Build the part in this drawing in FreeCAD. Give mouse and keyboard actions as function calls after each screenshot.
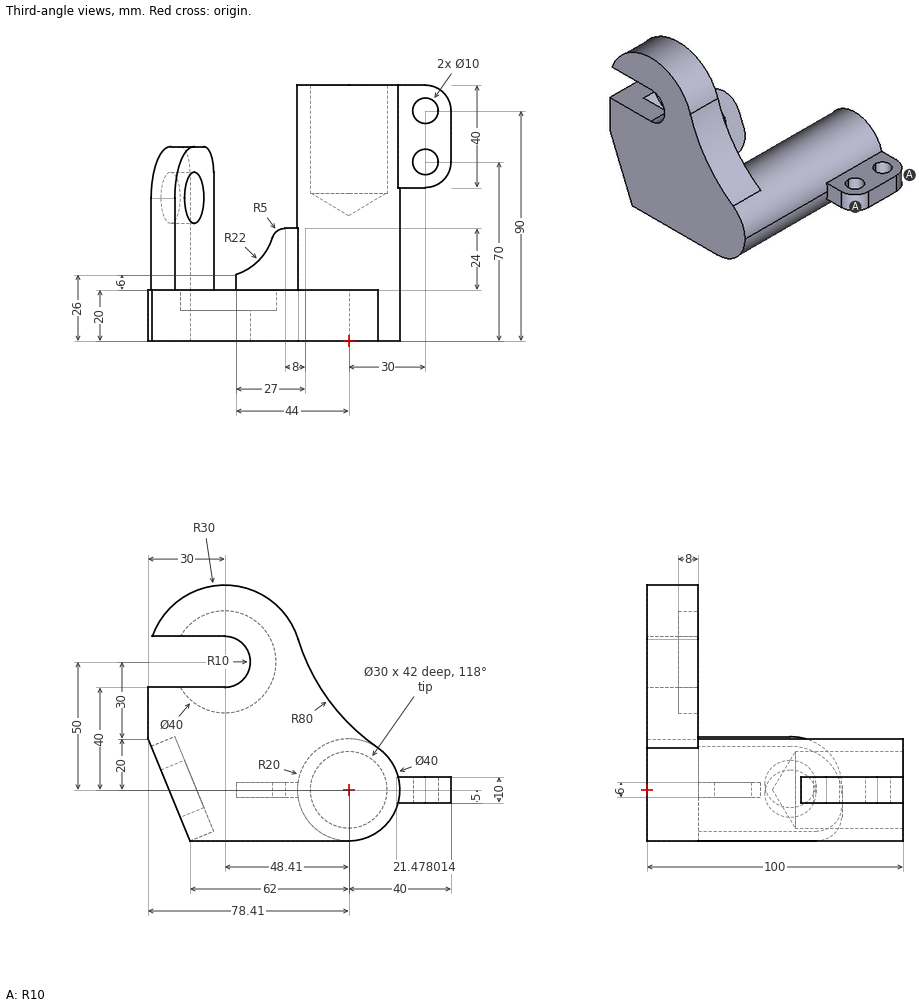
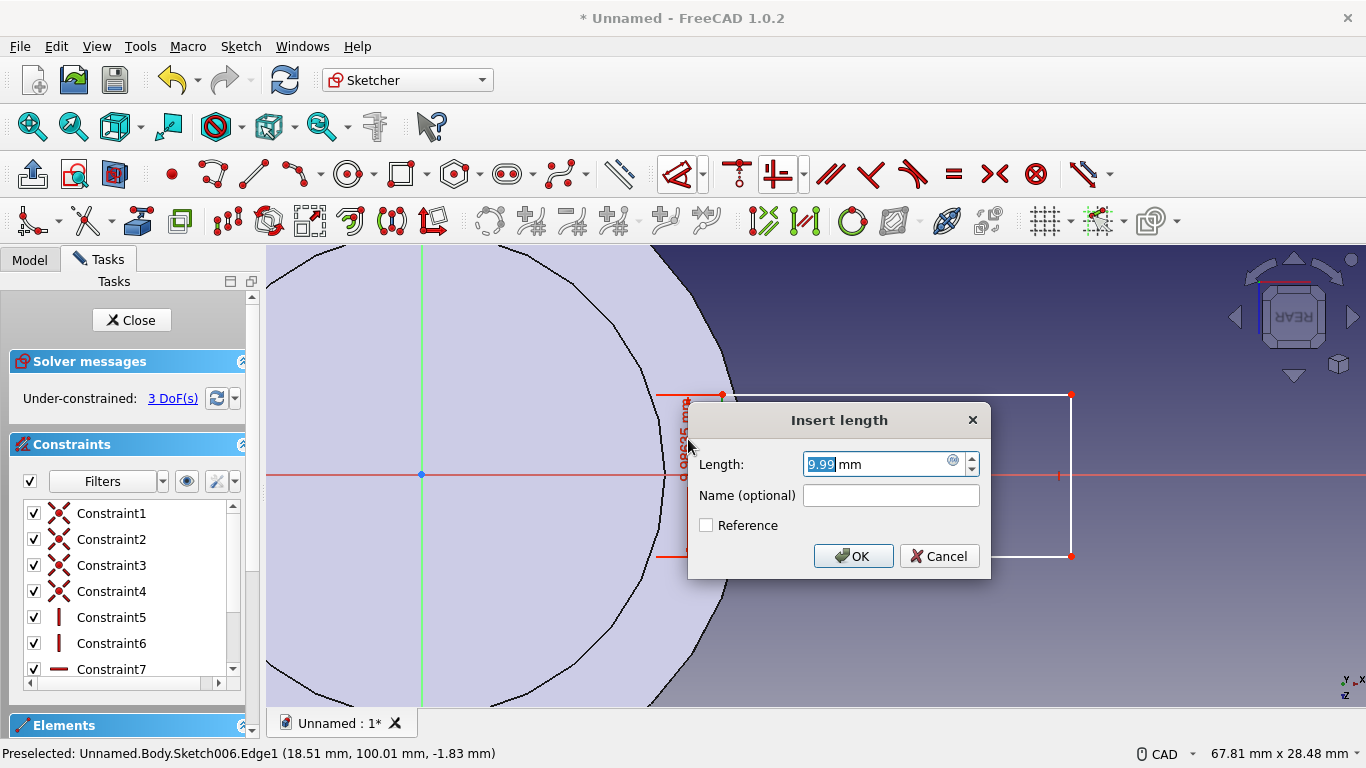
text(10)
key(Return)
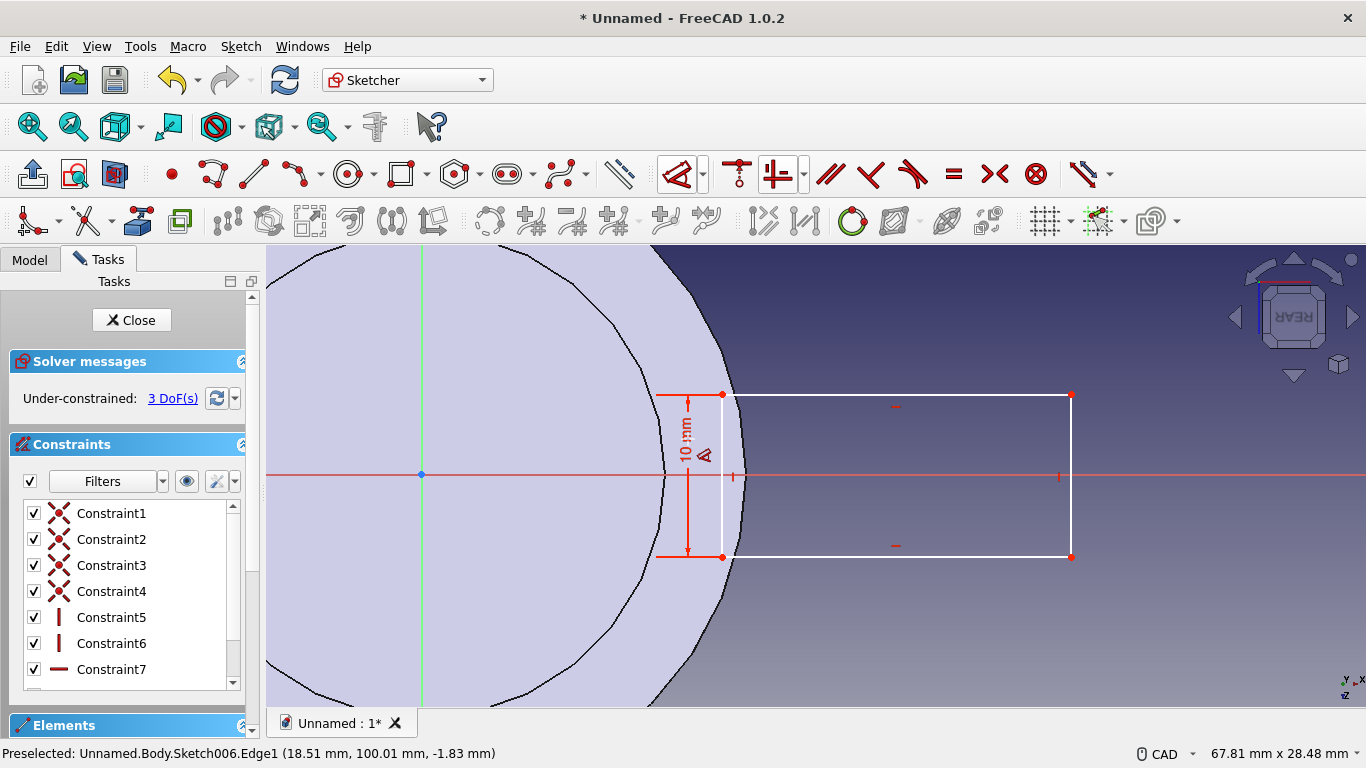
click(722, 395)
click(388, 435)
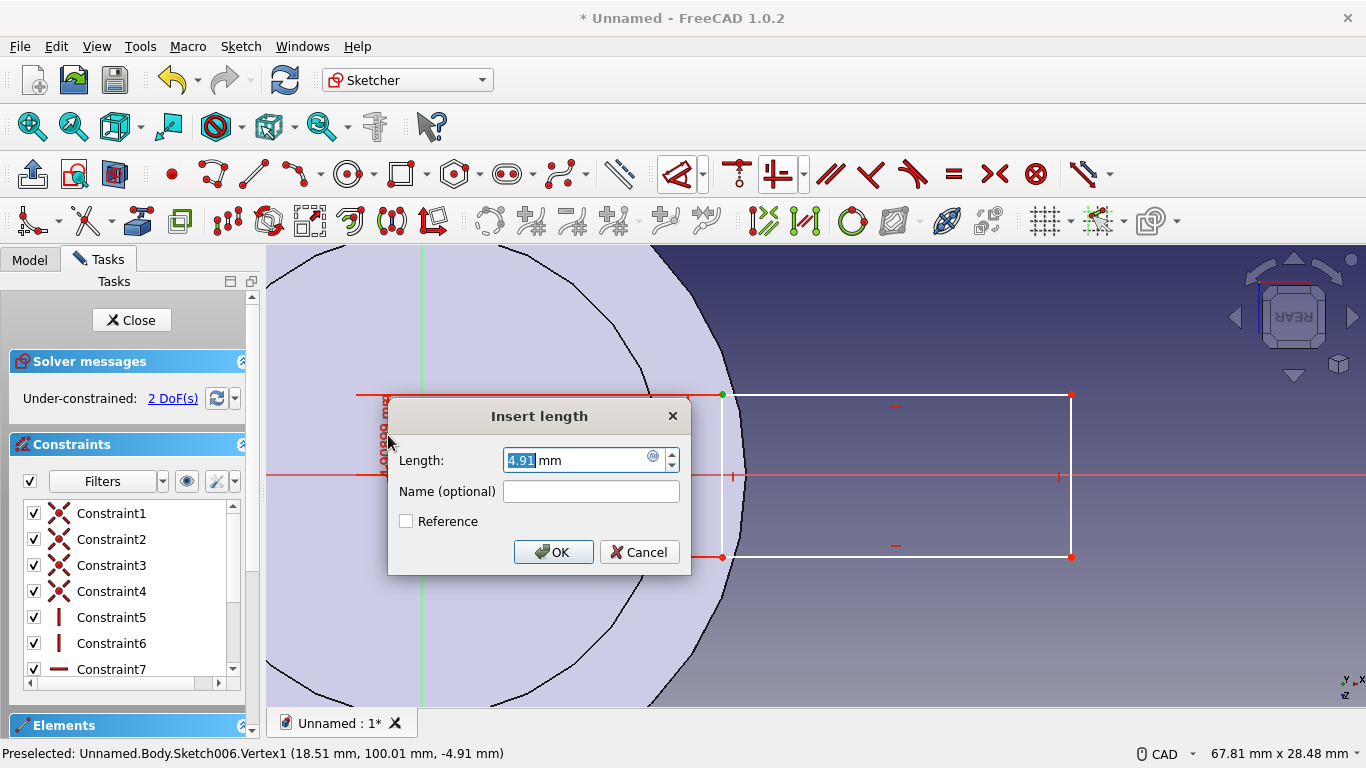
text(5)
key(Return)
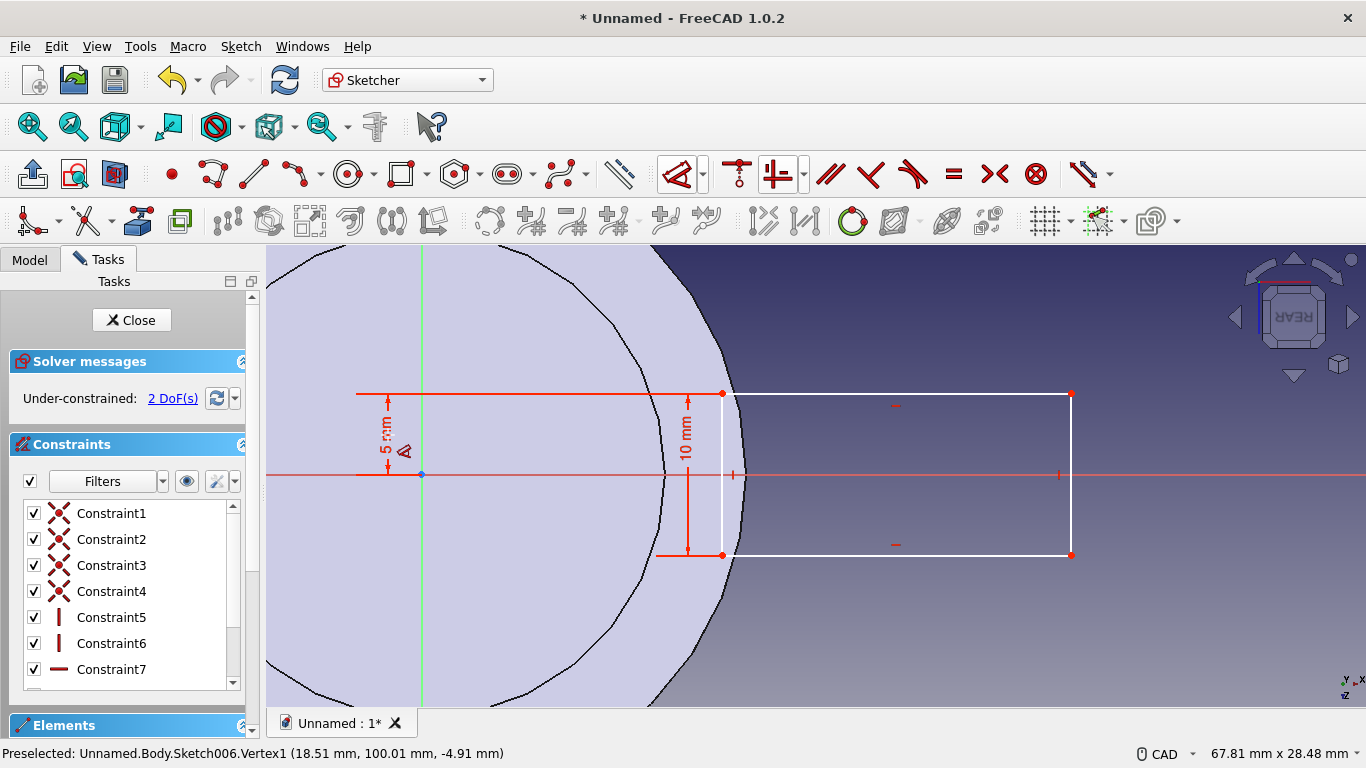
click(1071, 556)
click(746, 590)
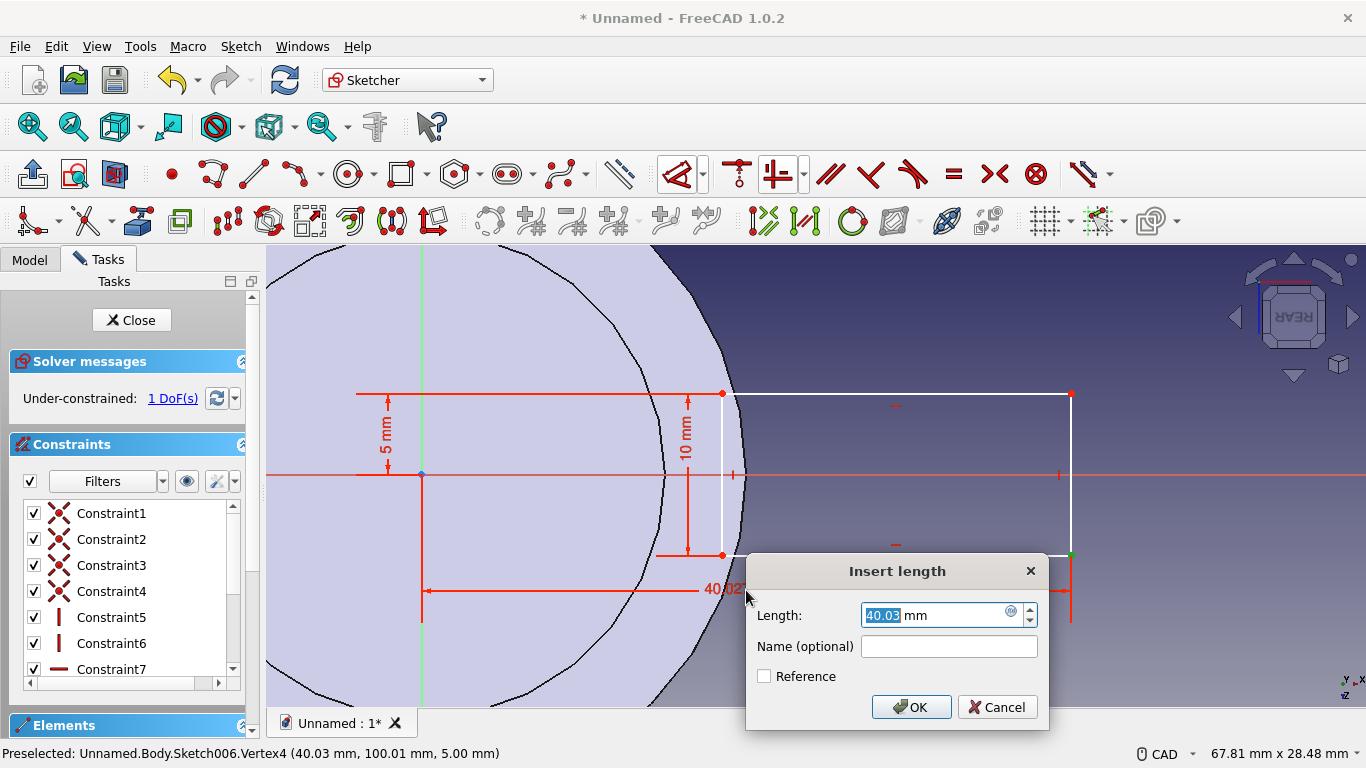
text(40)
key(Return)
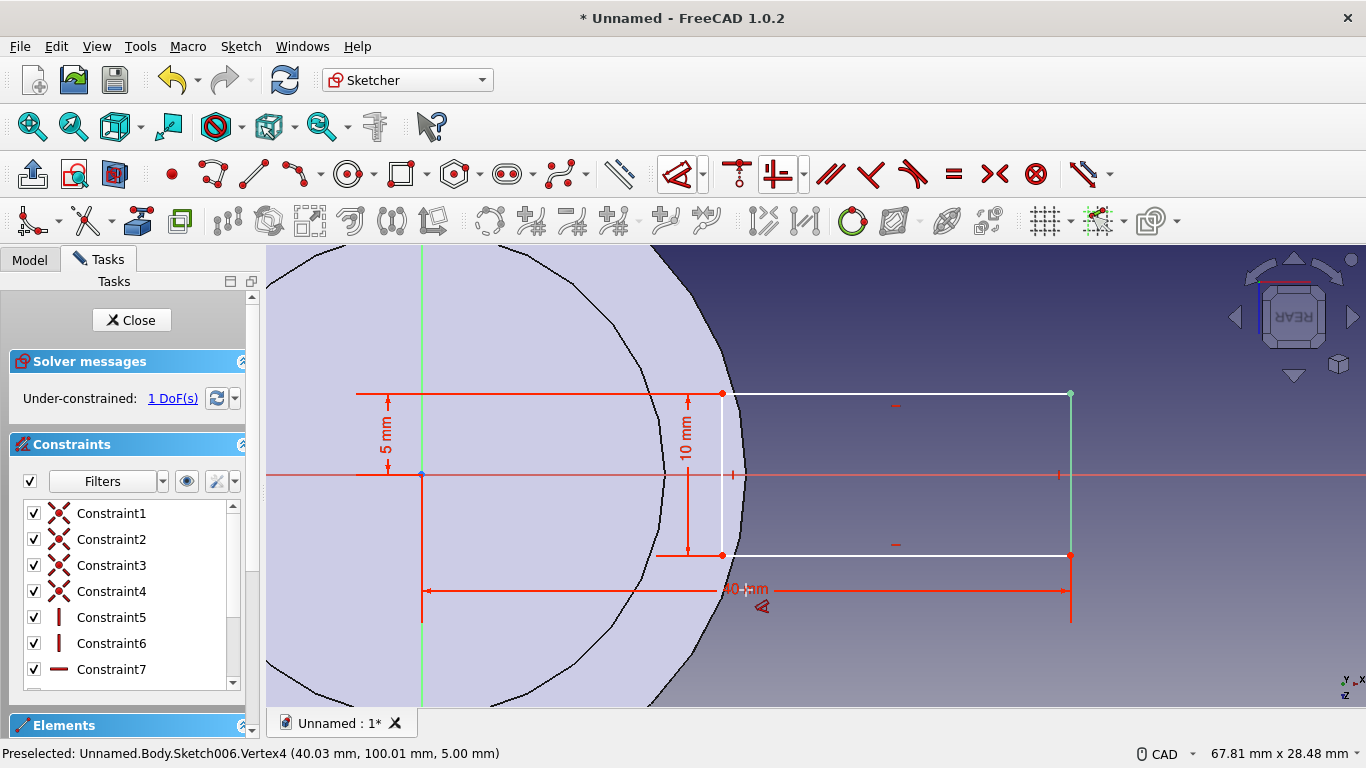
click(827, 556)
click(896, 590)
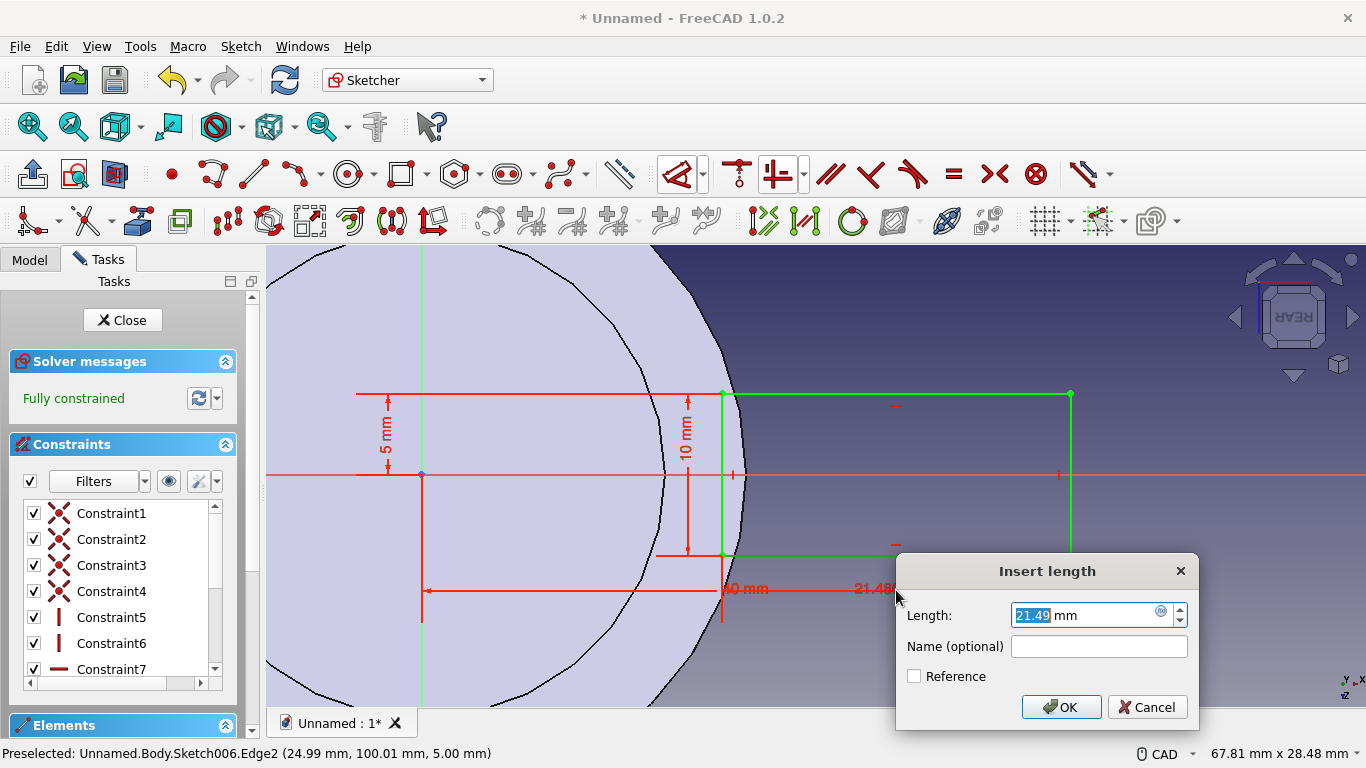
text(21.478014)
key(Return)
key(Escape)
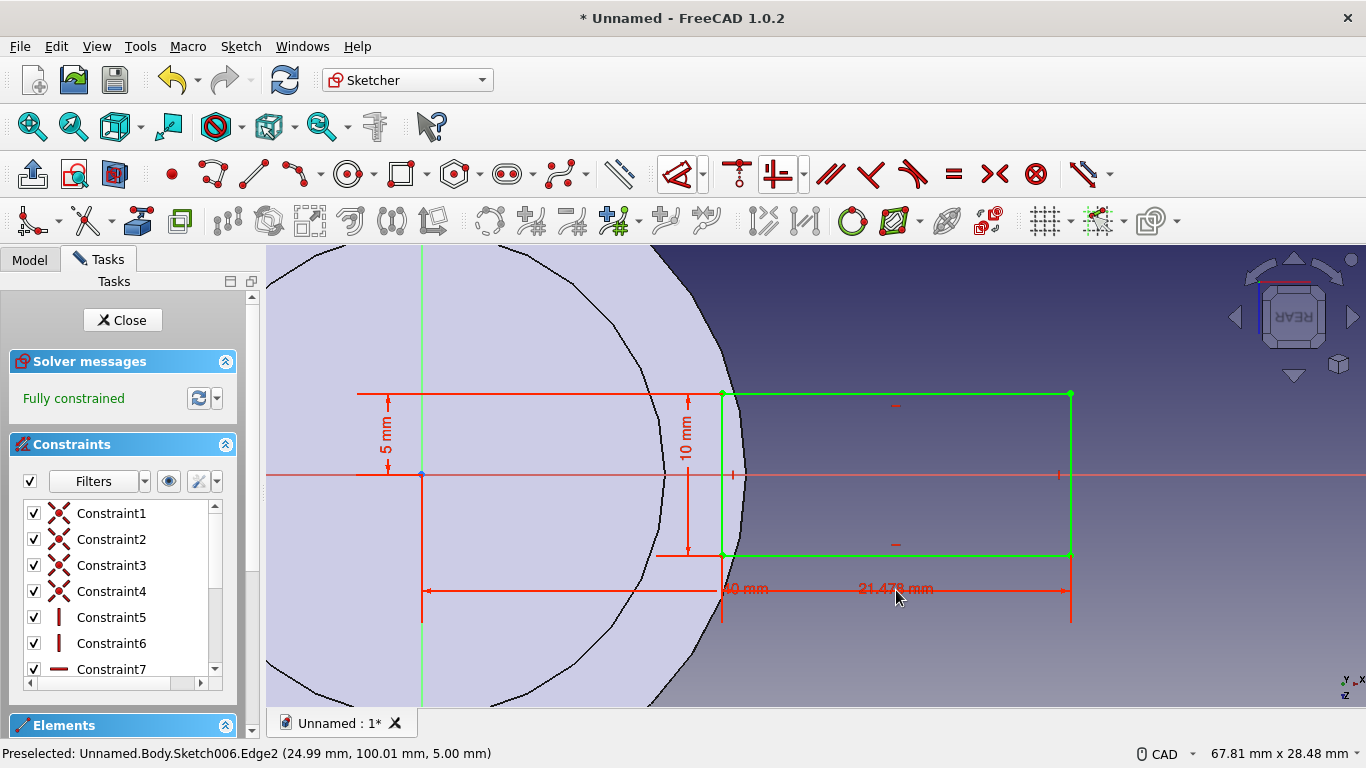
click(123, 320)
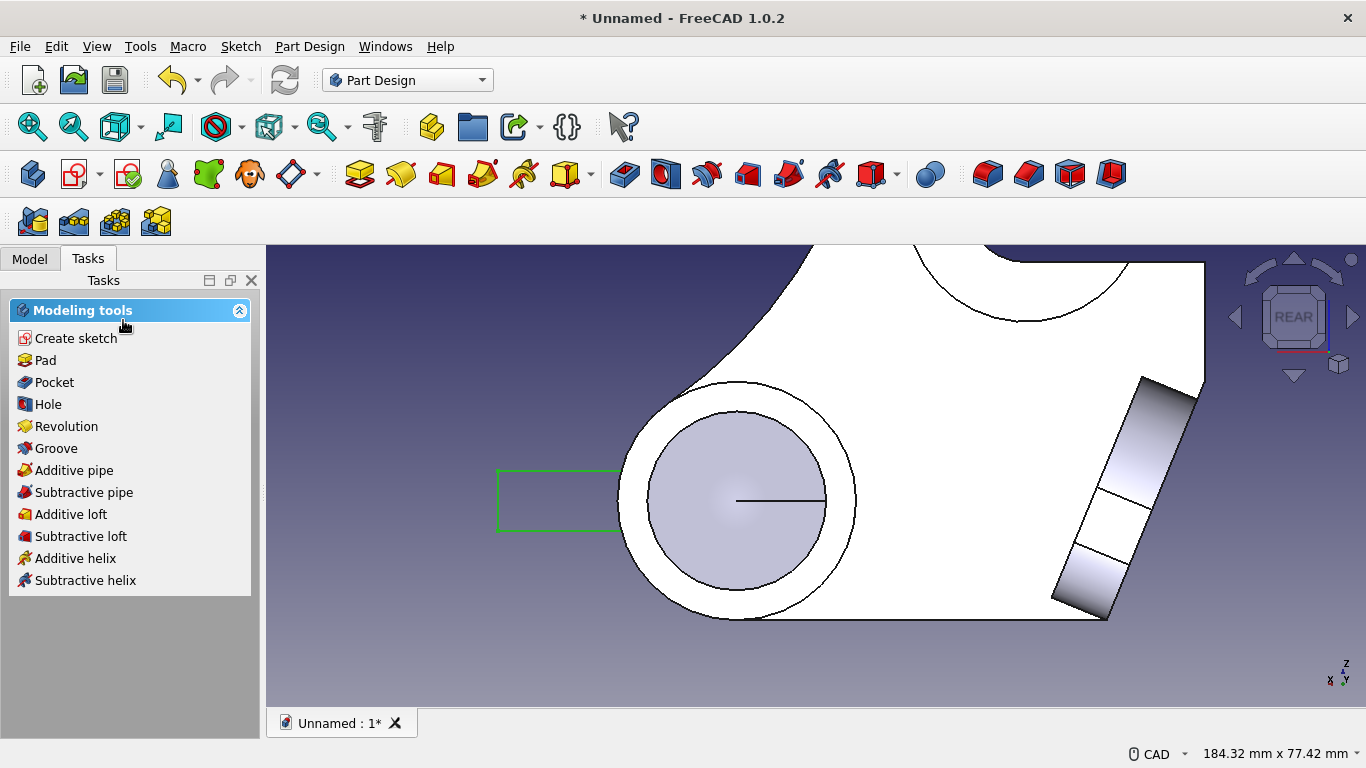
click(360, 174)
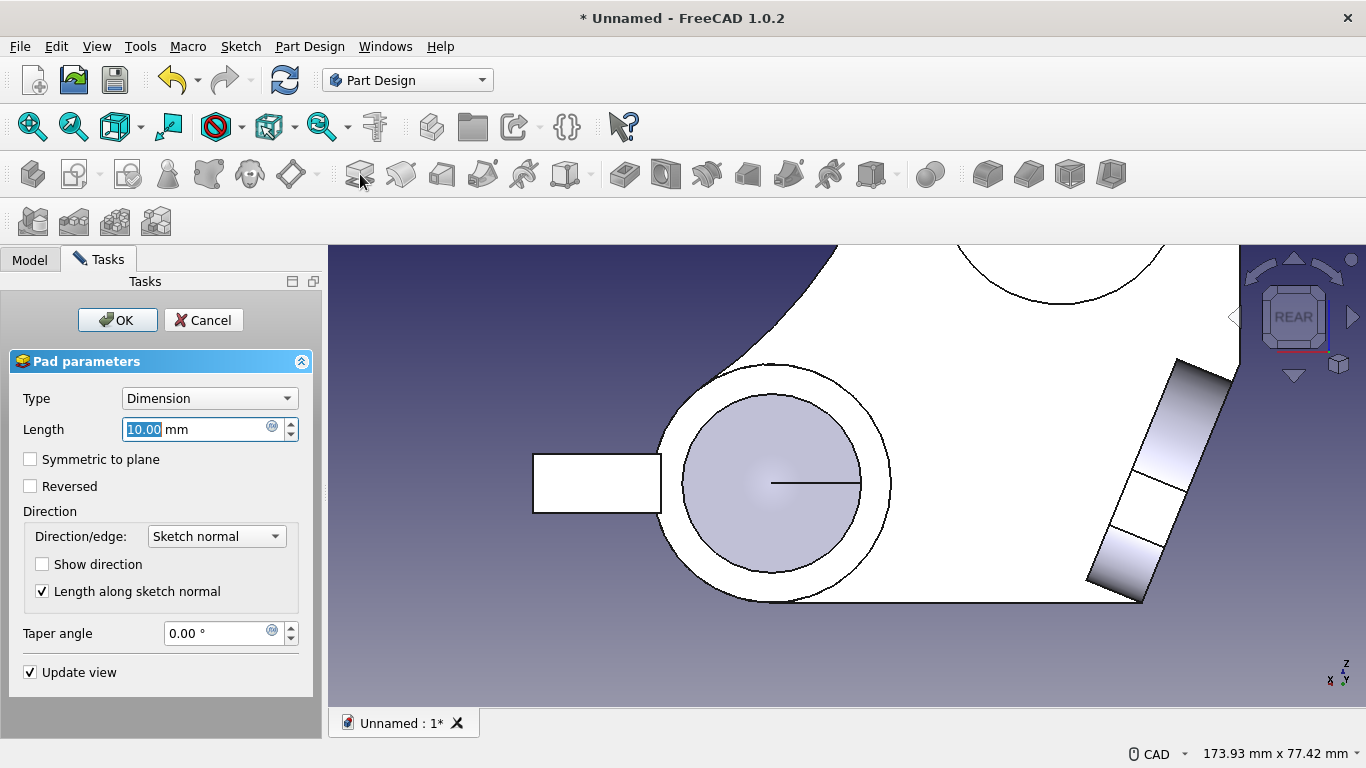
text(40)
key(Tab)